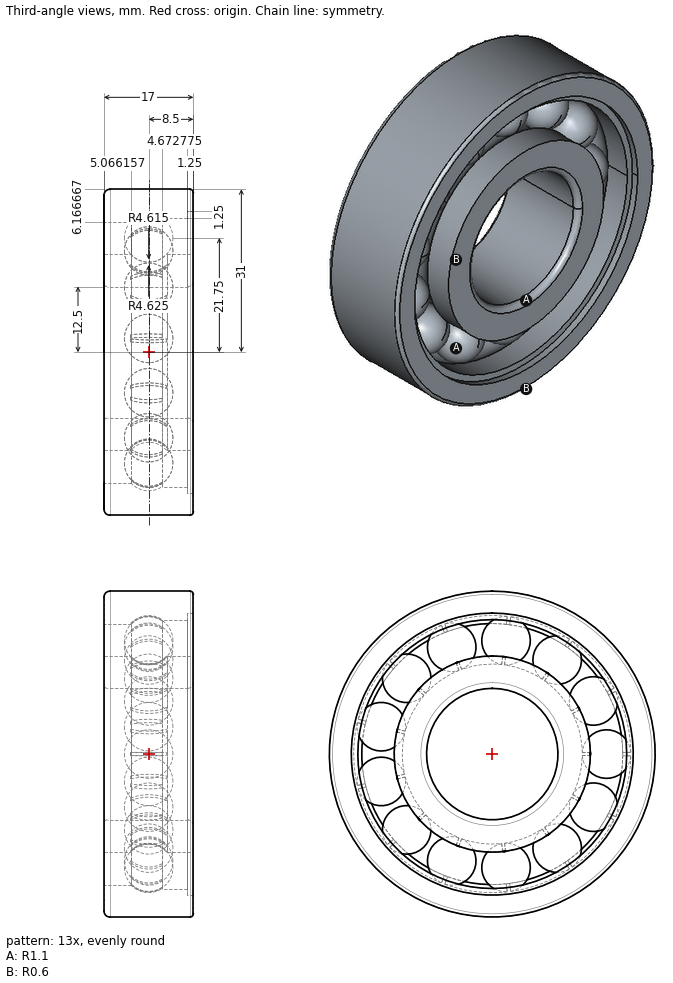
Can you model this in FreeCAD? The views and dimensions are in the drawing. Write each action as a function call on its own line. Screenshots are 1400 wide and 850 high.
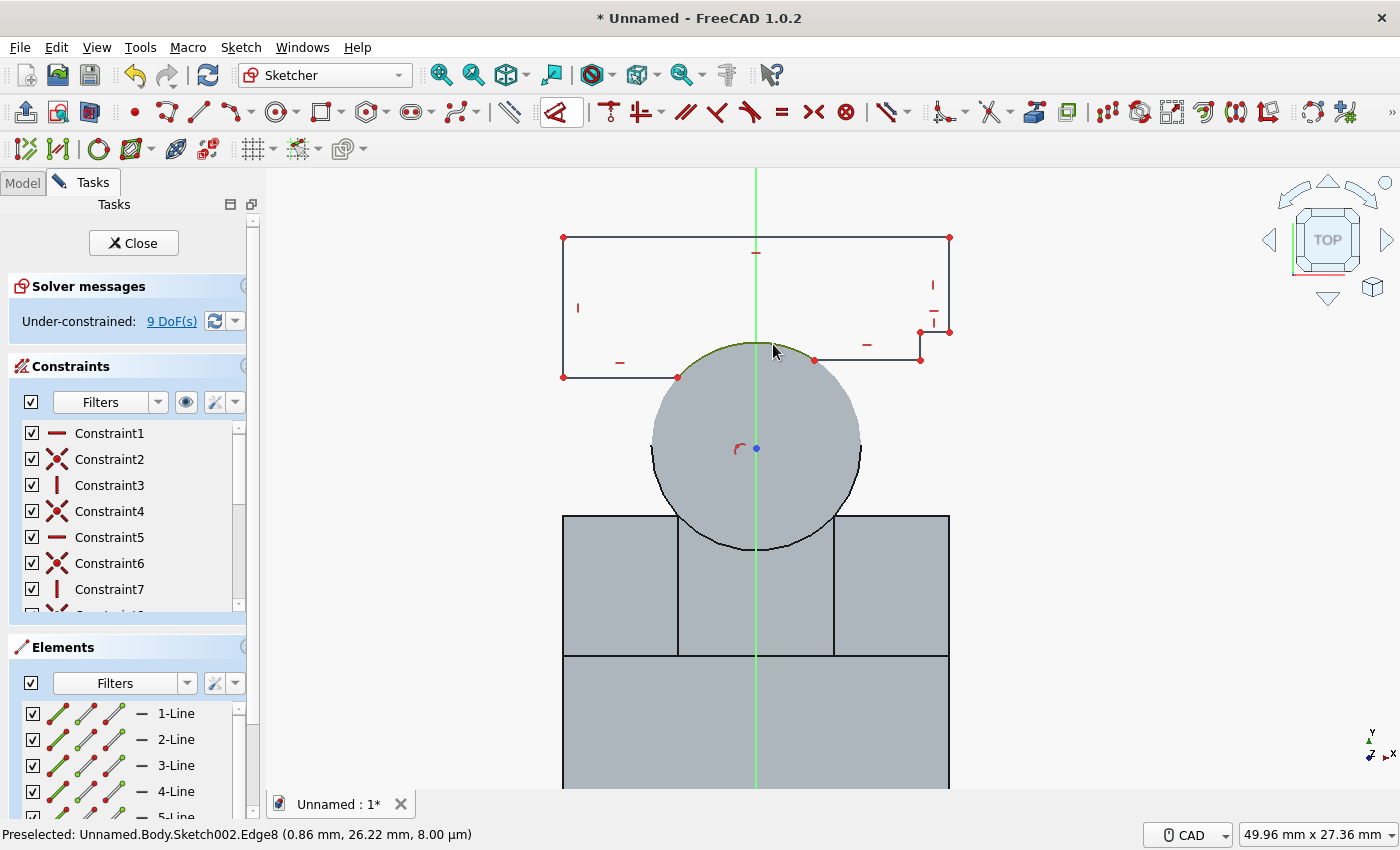
click(578, 112)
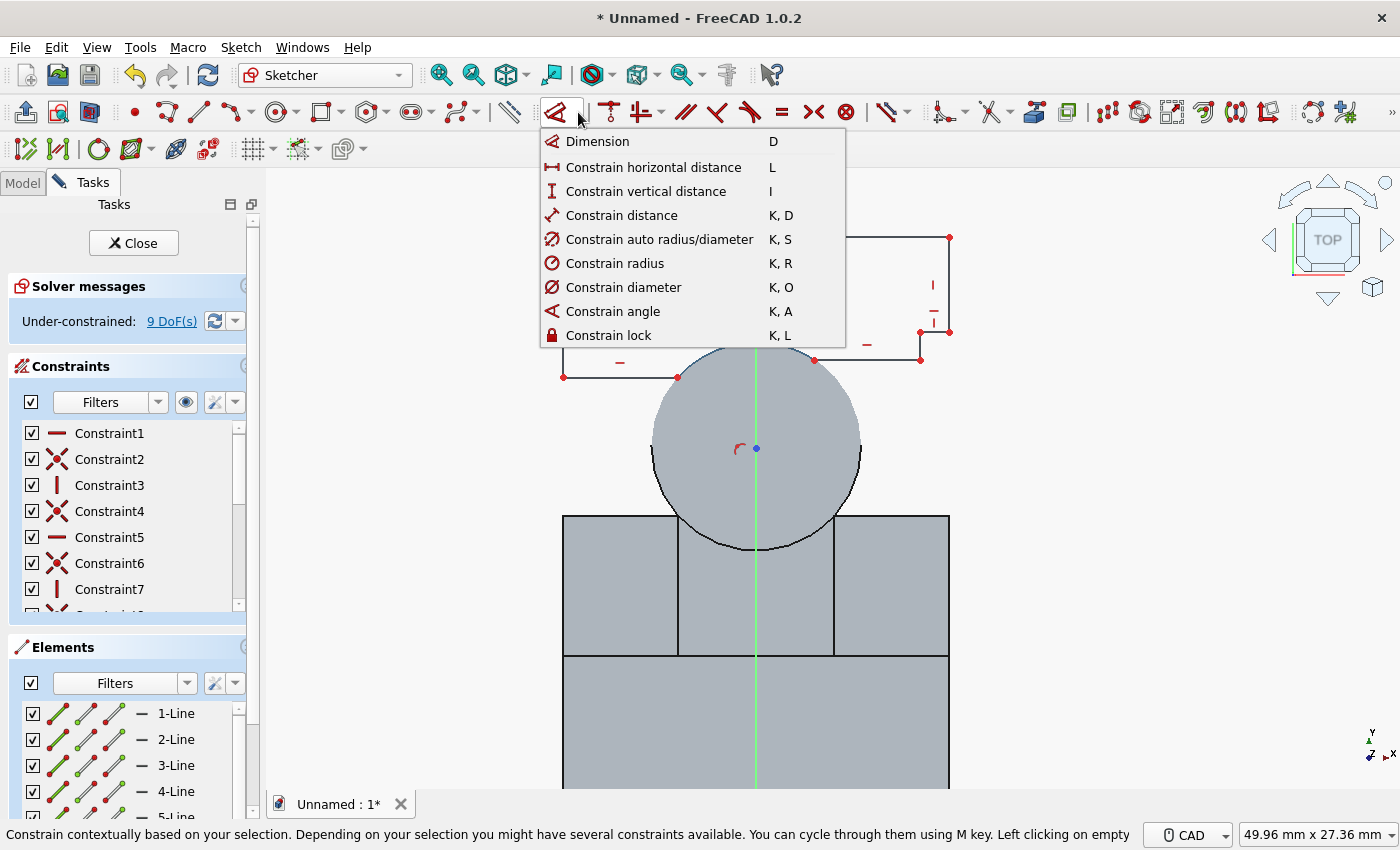
click(693, 263)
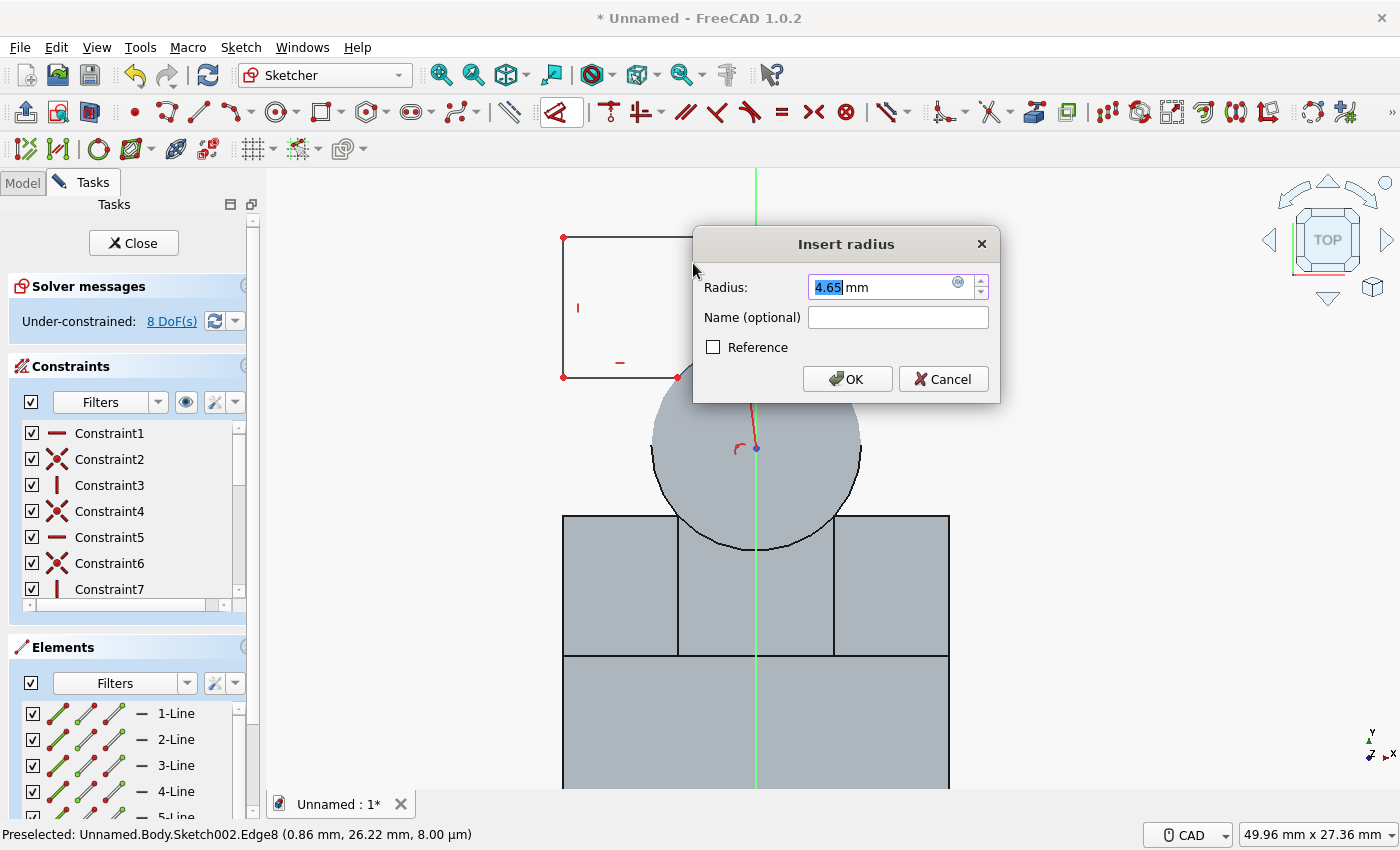
text(4.615)
key(Return)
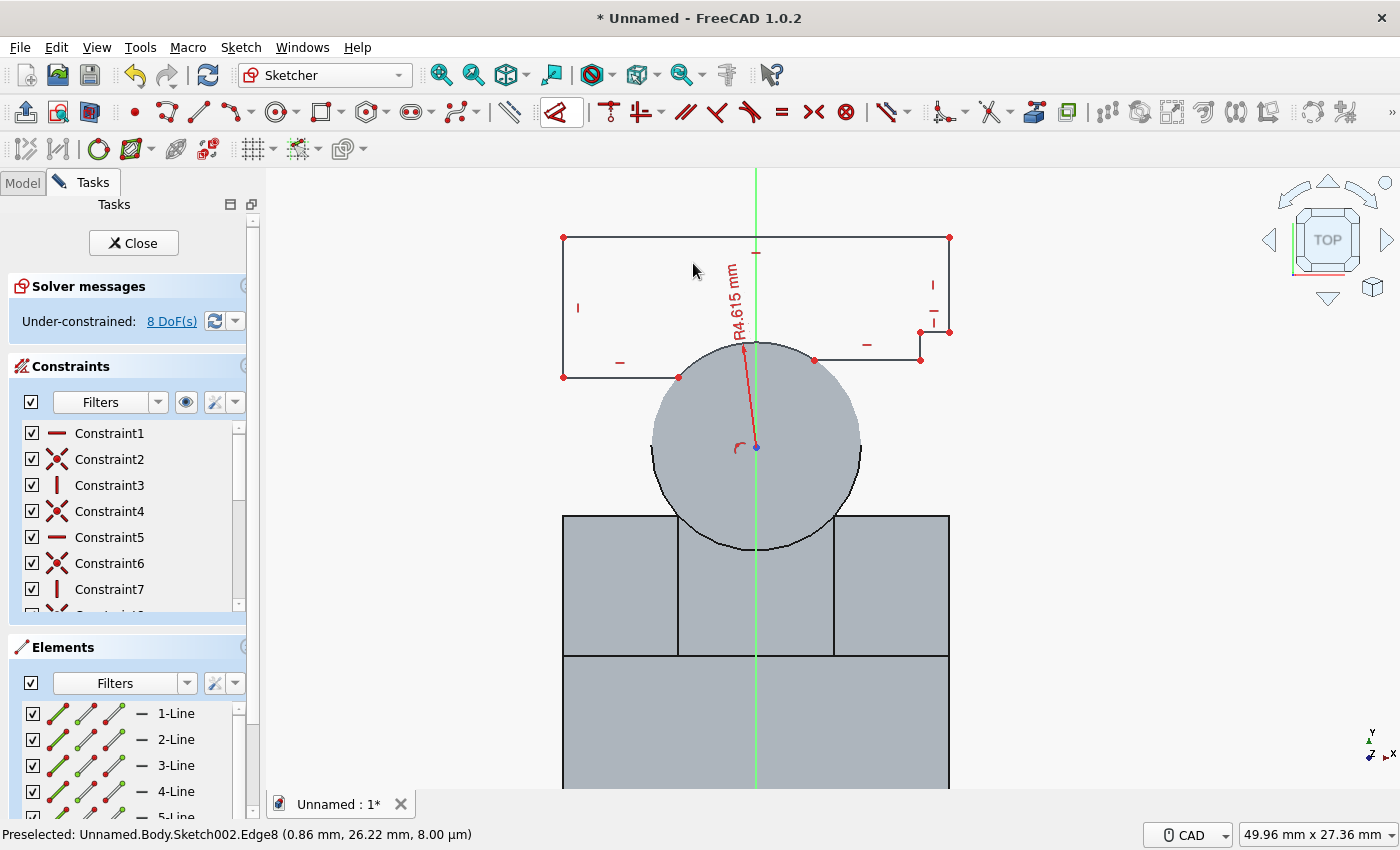
click(833, 237)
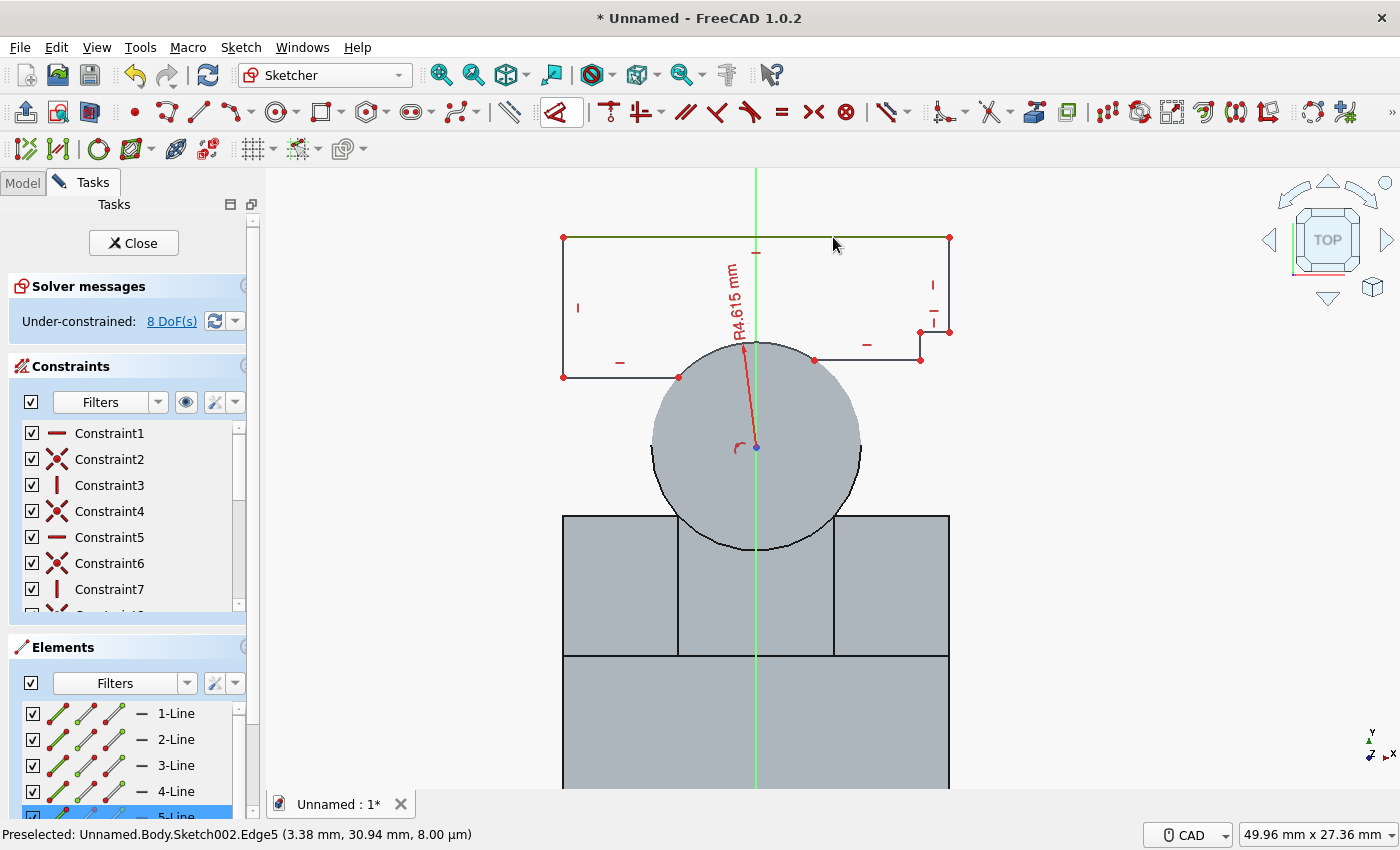
click(578, 112)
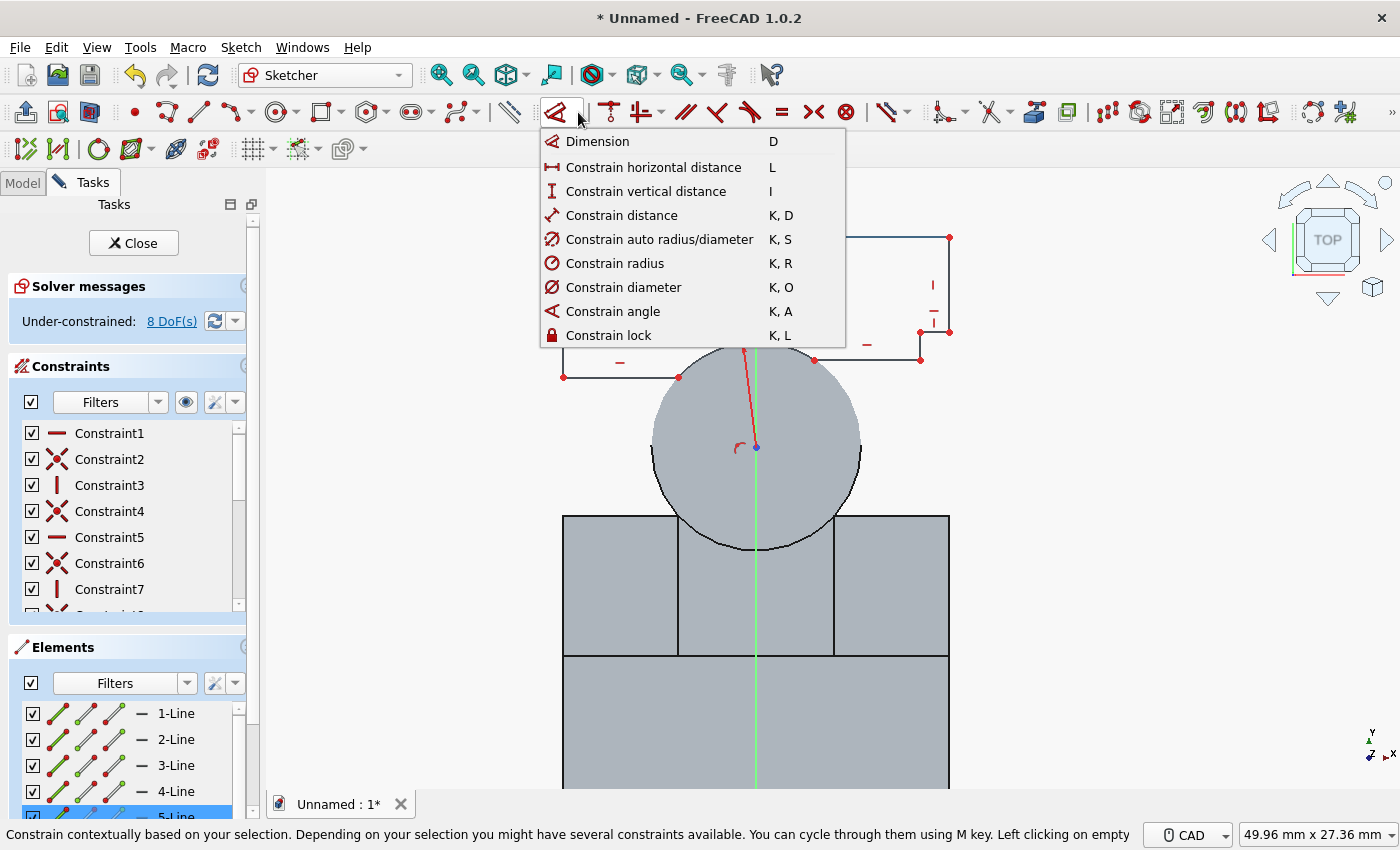
click(693, 167)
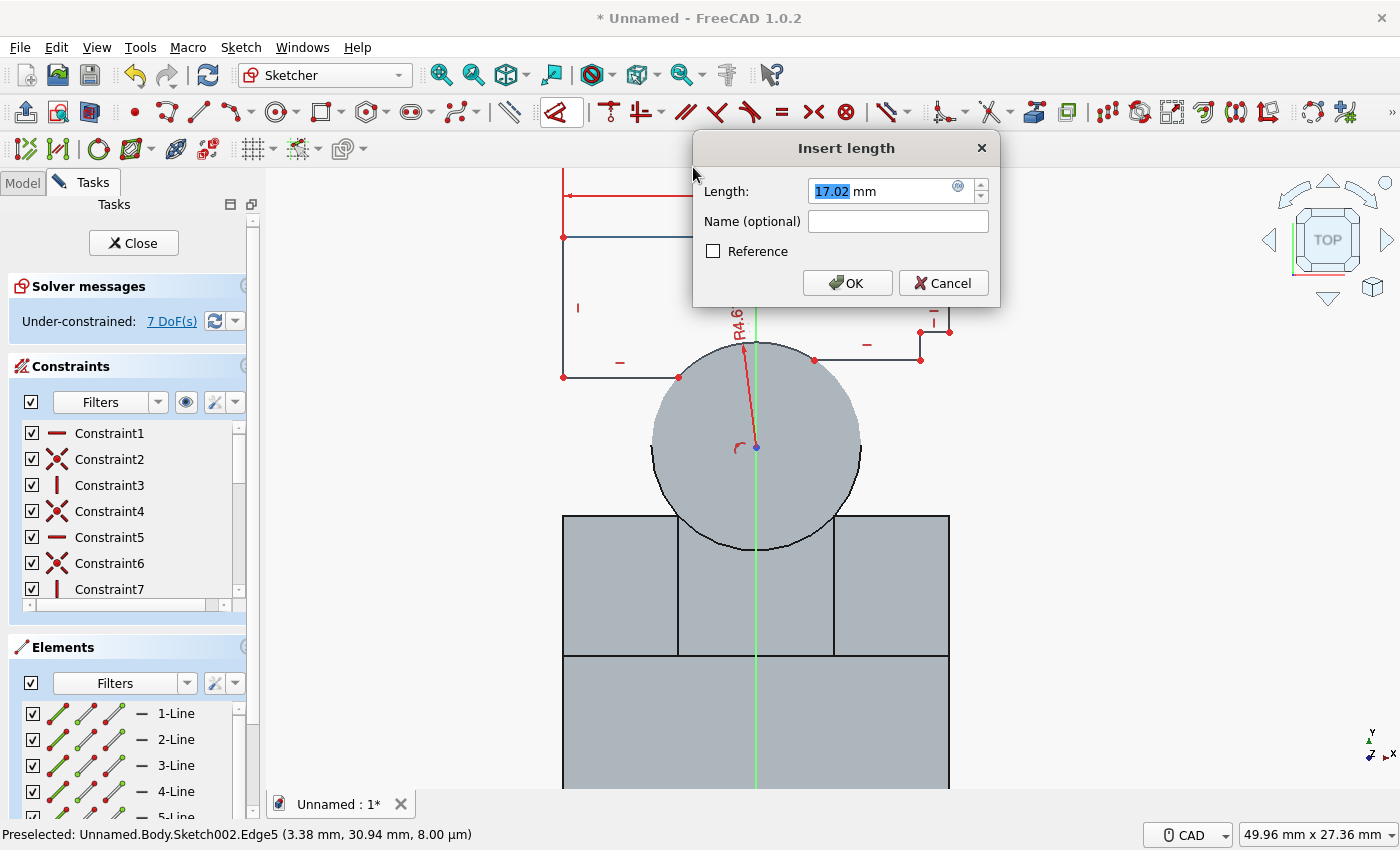
text(17)
key(Return)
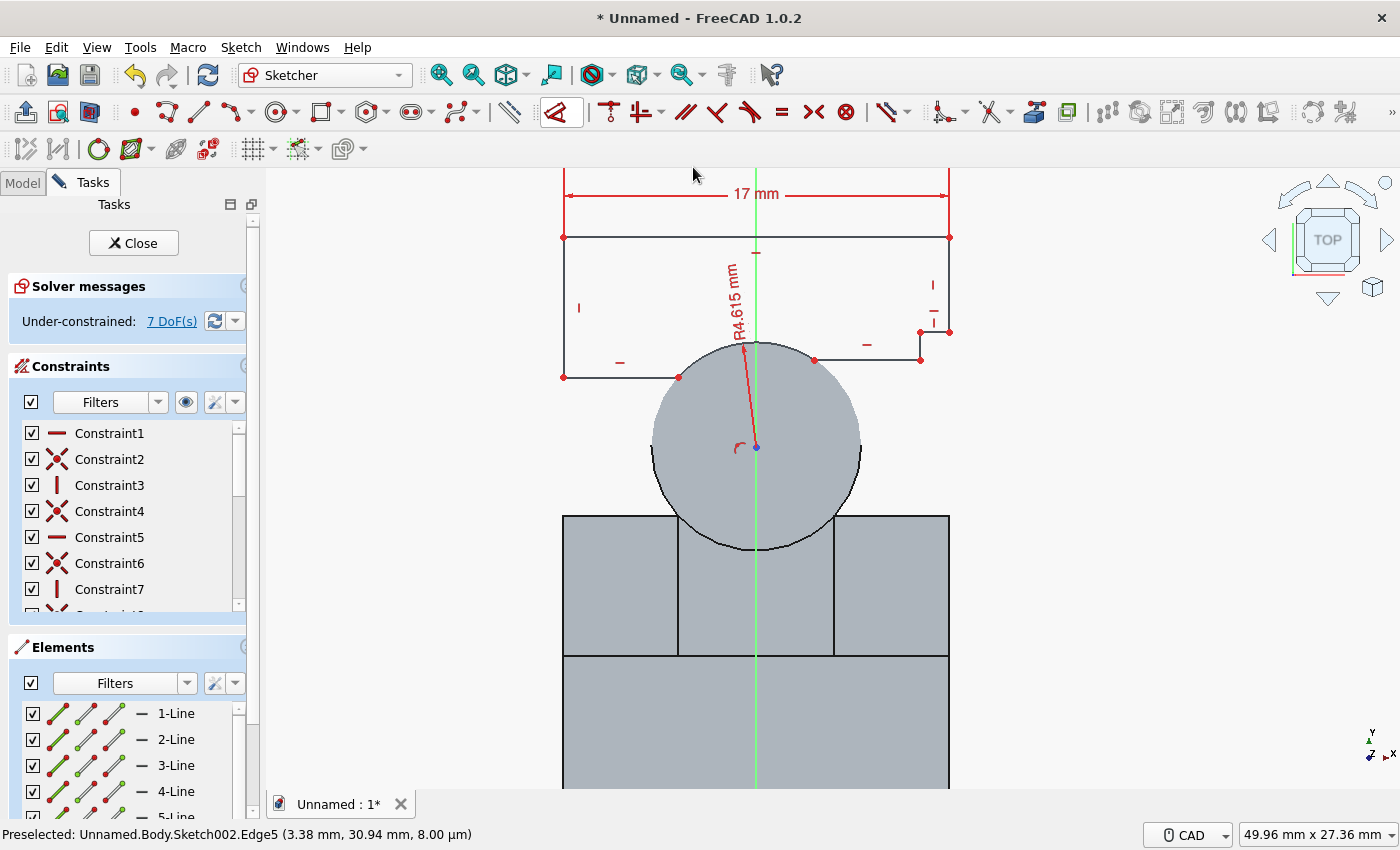
click(949, 237)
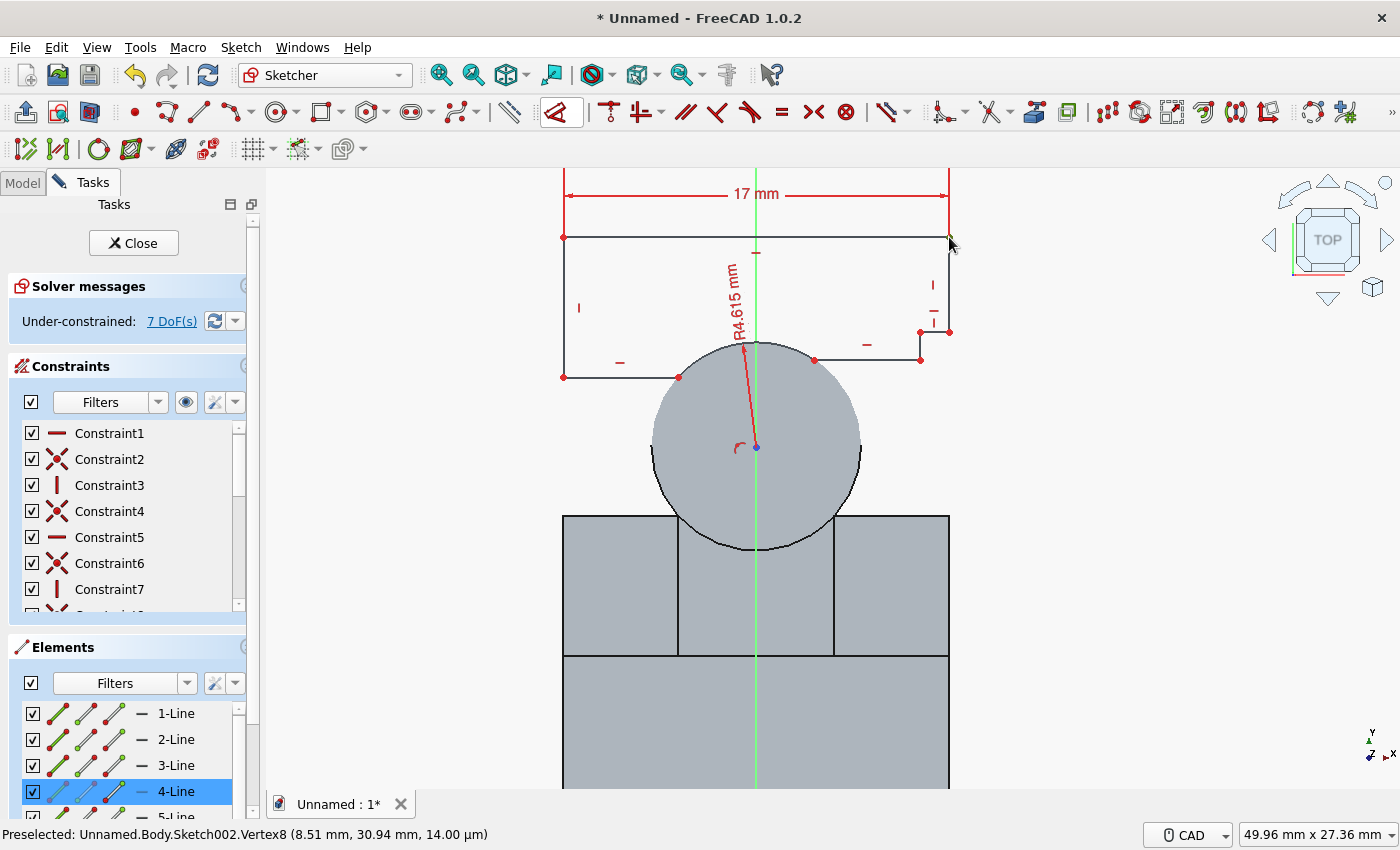
key(i)